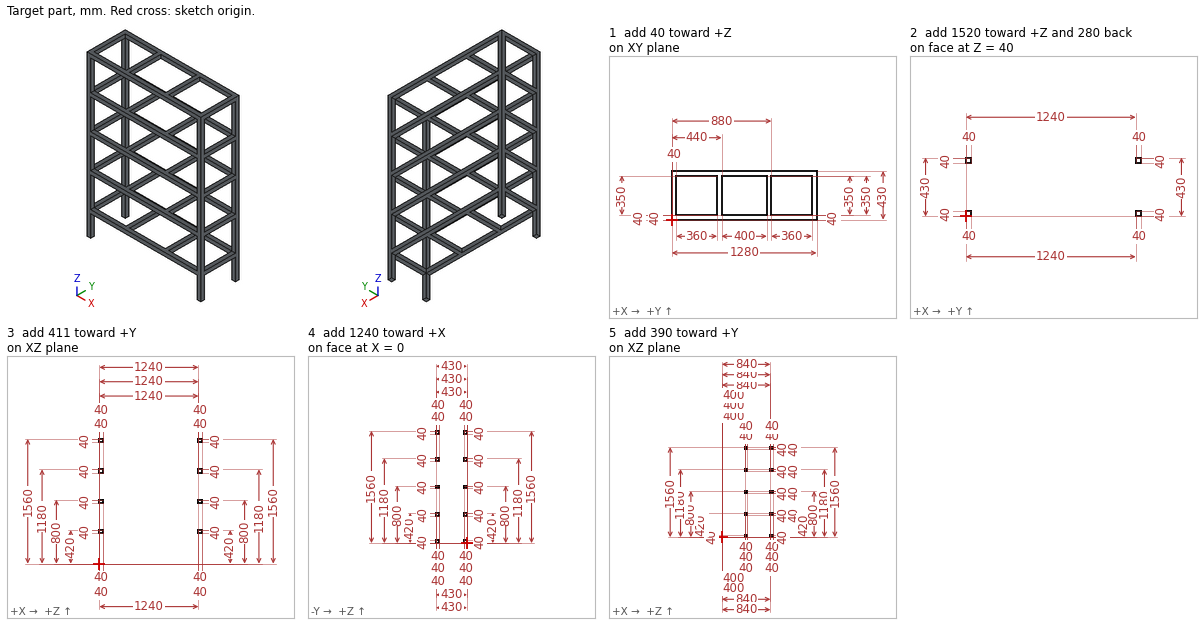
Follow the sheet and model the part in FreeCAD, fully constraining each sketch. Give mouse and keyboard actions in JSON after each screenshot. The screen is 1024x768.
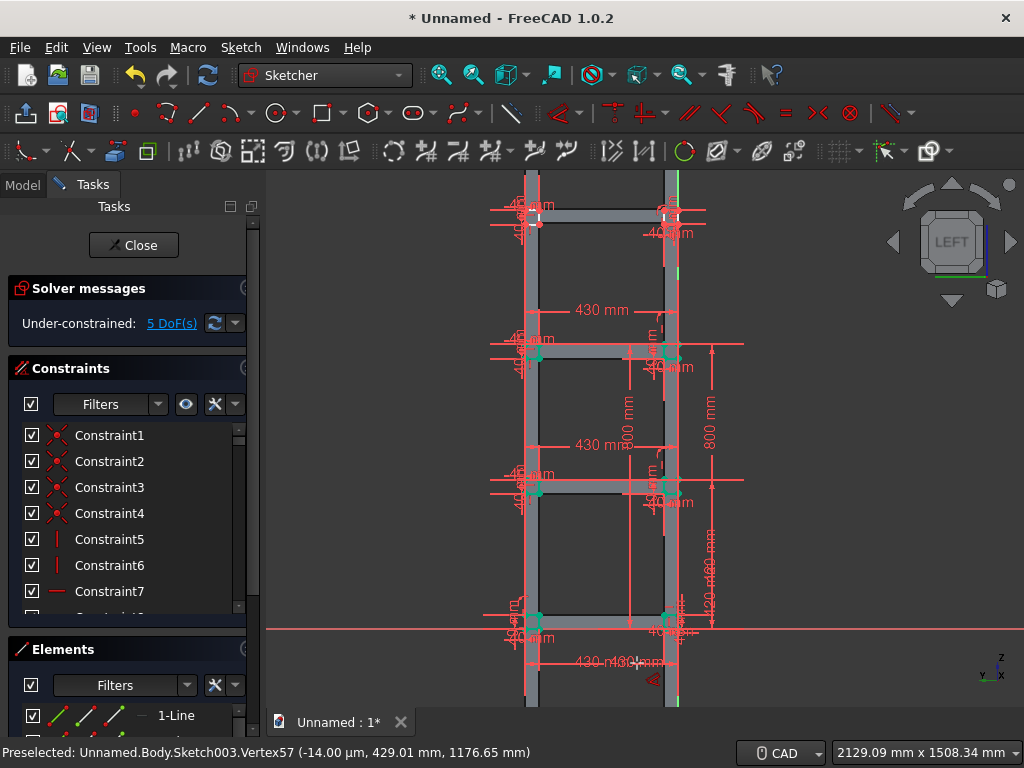
{"action": "scroll", "coordinate": [525, 615], "scroll_direction": "down", "scroll_amount": 2}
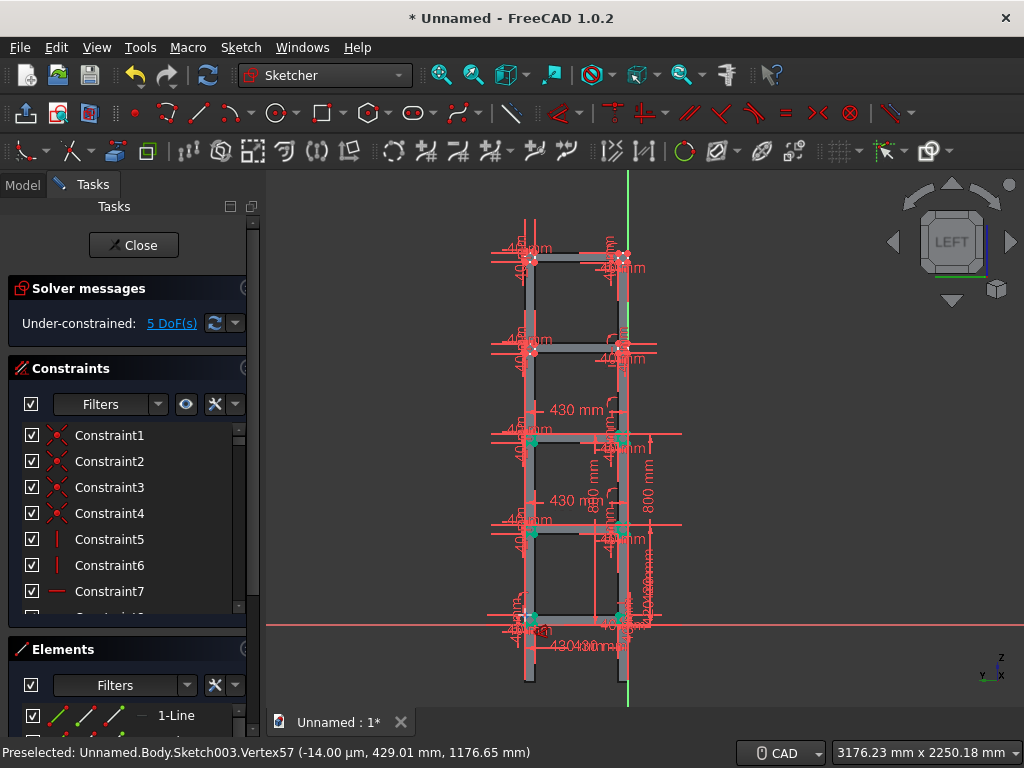
{"action": "scroll", "coordinate": [525, 253], "scroll_direction": "up", "scroll_amount": 2}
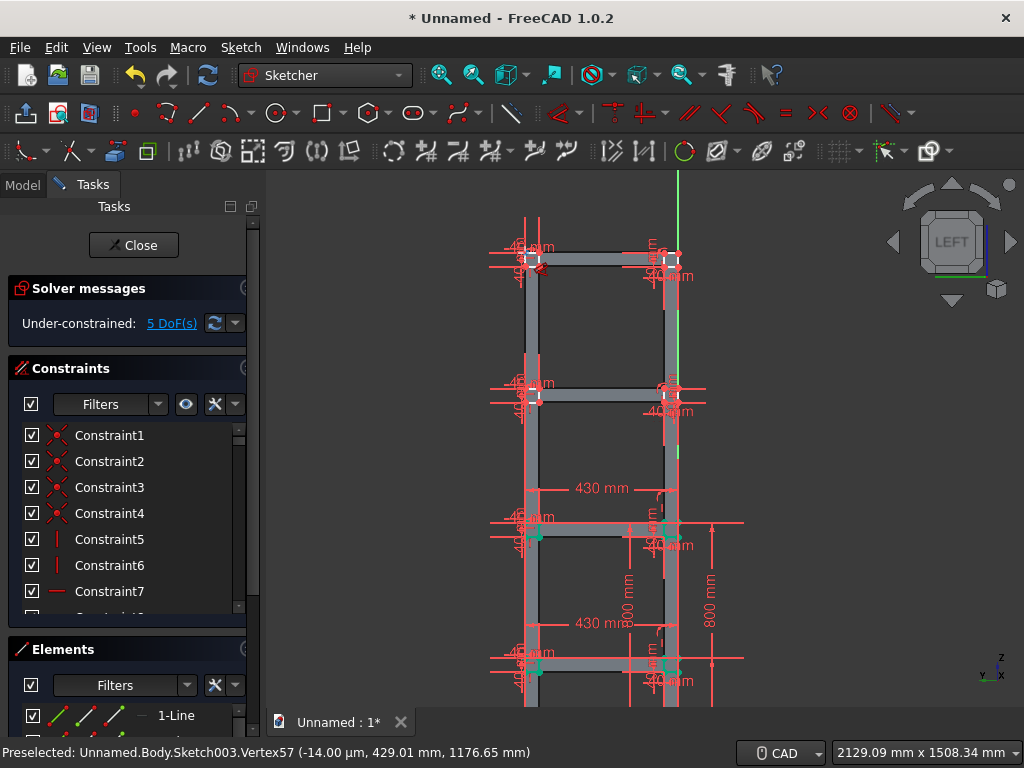
{"action": "left_click", "coordinate": [525, 253]}
{"action": "left_click", "coordinate": [602, 219]}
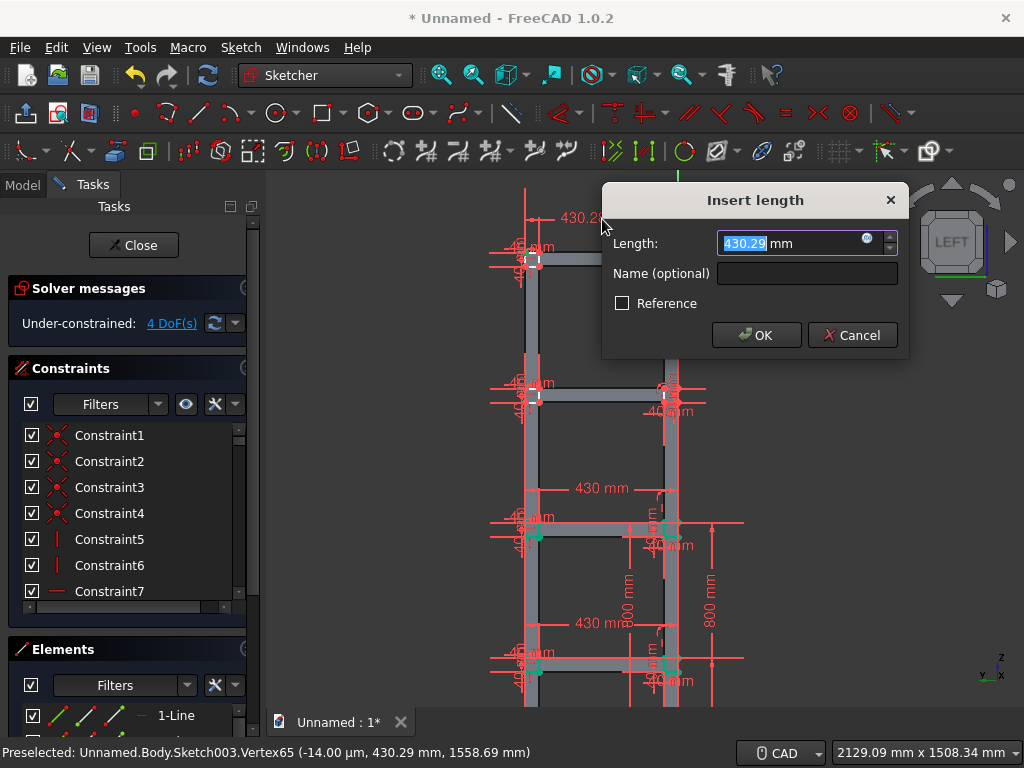
{"action": "type", "text": "430"}
{"action": "key", "text": "Return"}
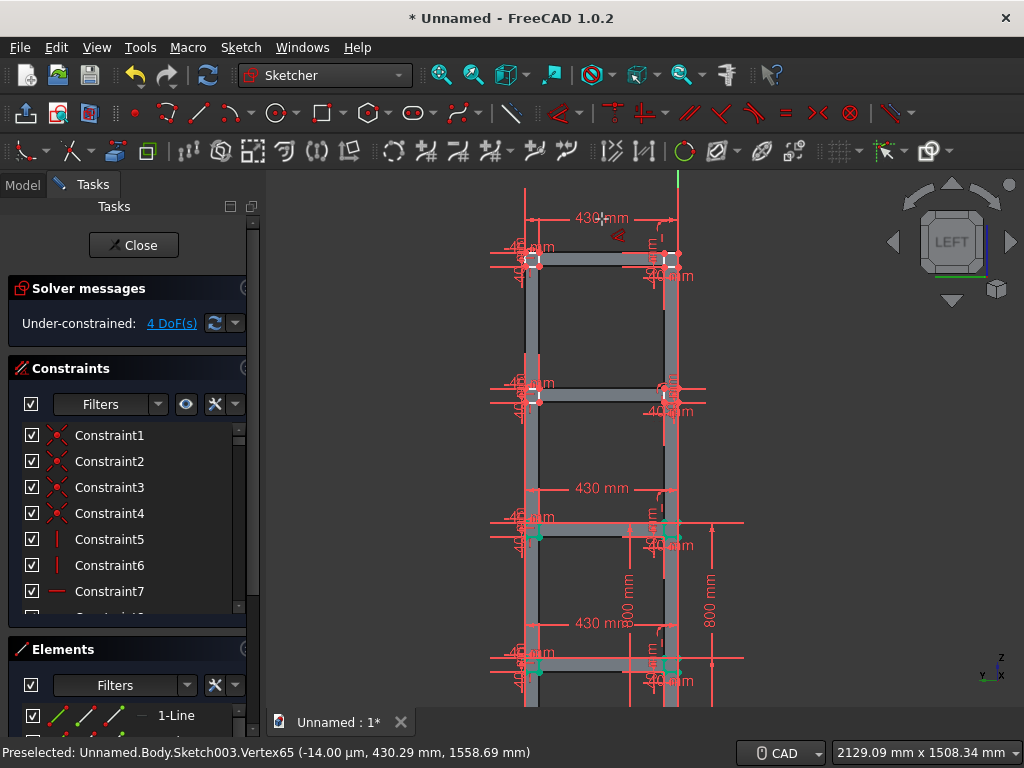
{"action": "left_click", "coordinate": [664, 389]}
{"action": "left_click", "coordinate": [712, 467]}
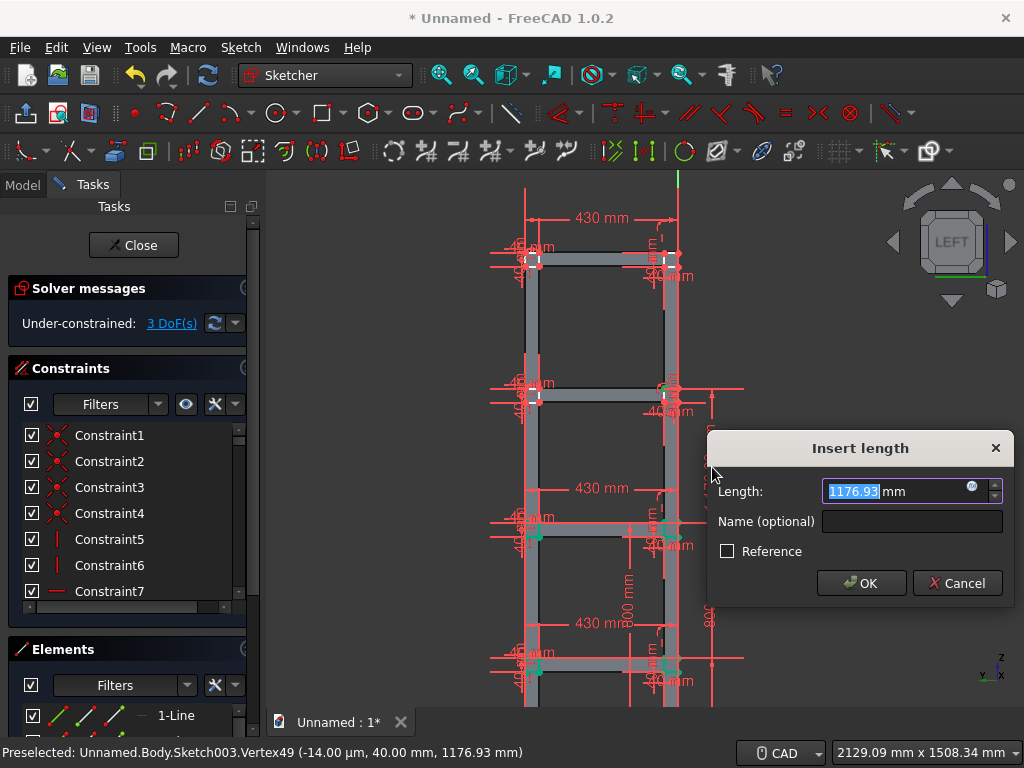
{"action": "type", "text": "1180"}
{"action": "key", "text": "Return"}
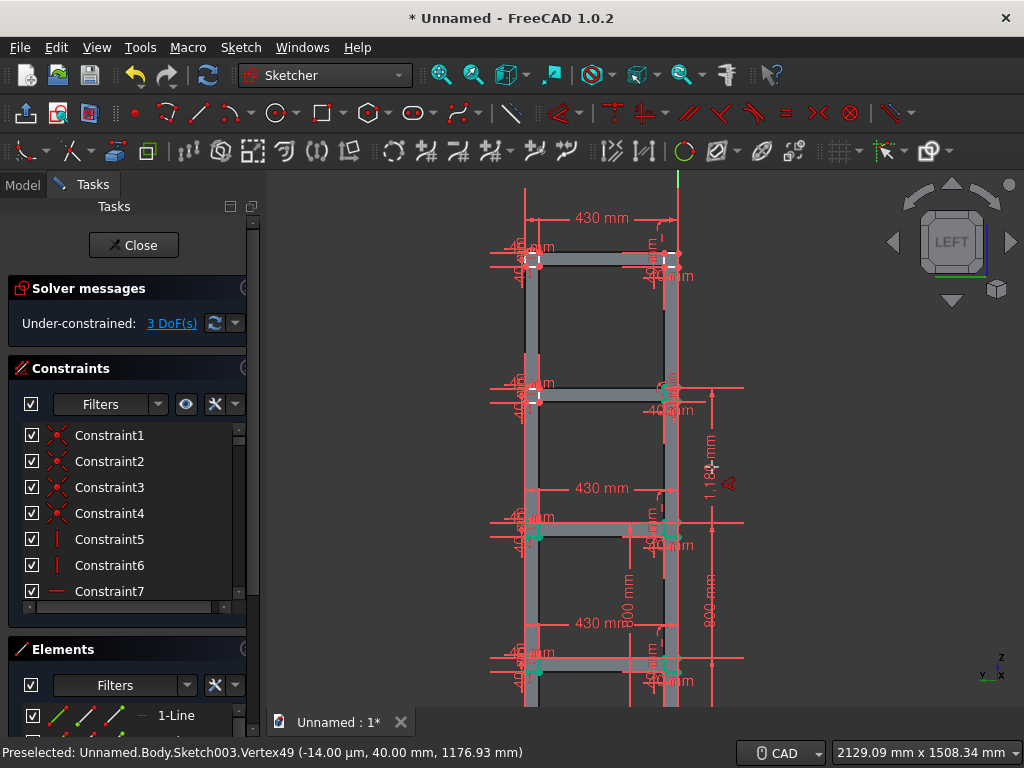
{"action": "left_click", "coordinate": [525, 389]}
{"action": "left_click", "coordinate": [712, 635]}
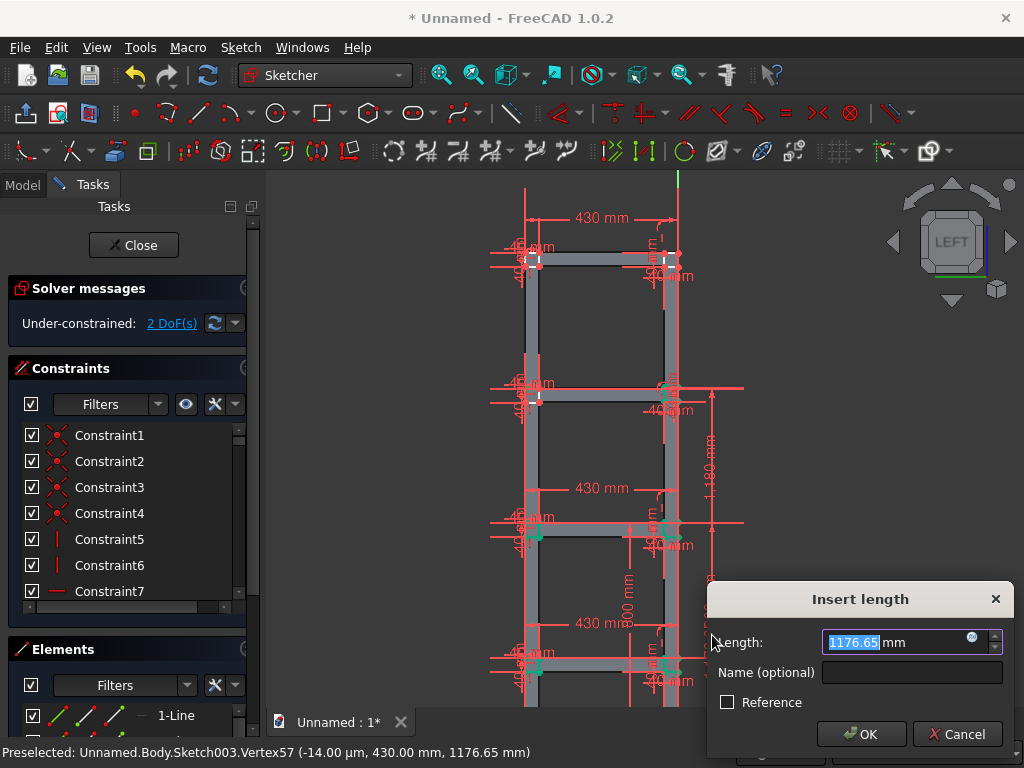
{"action": "type", "text": "1180"}
{"action": "key", "text": "Return"}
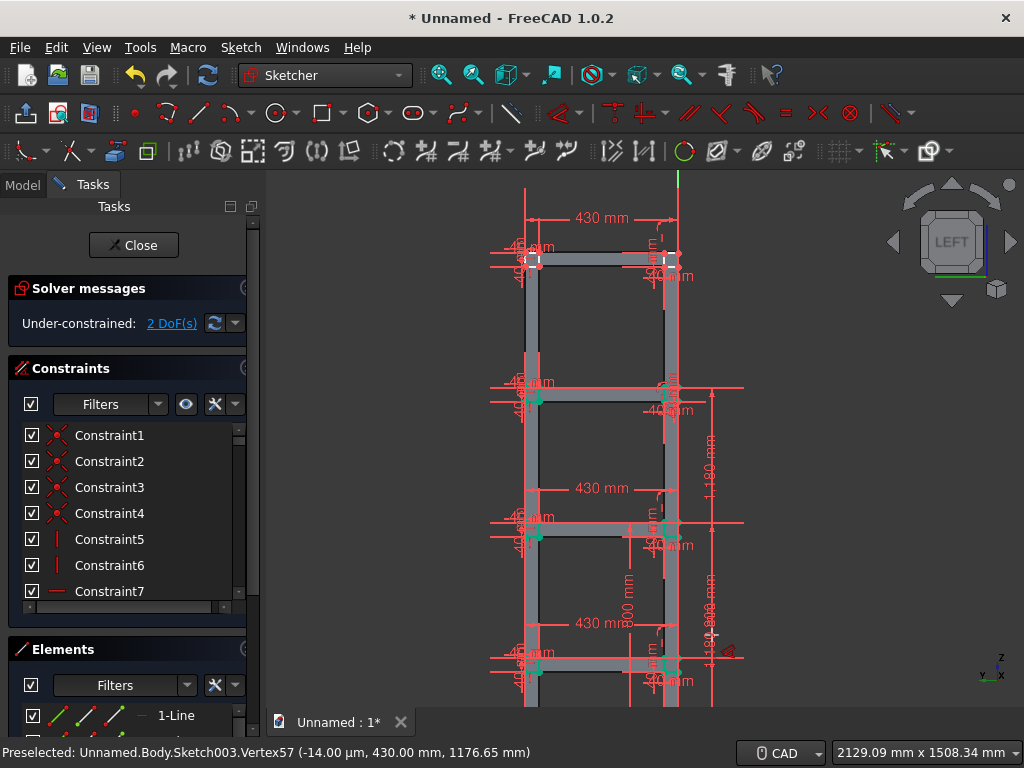
{"action": "left_click", "coordinate": [525, 253]}
{"action": "left_click", "coordinate": [712, 368]}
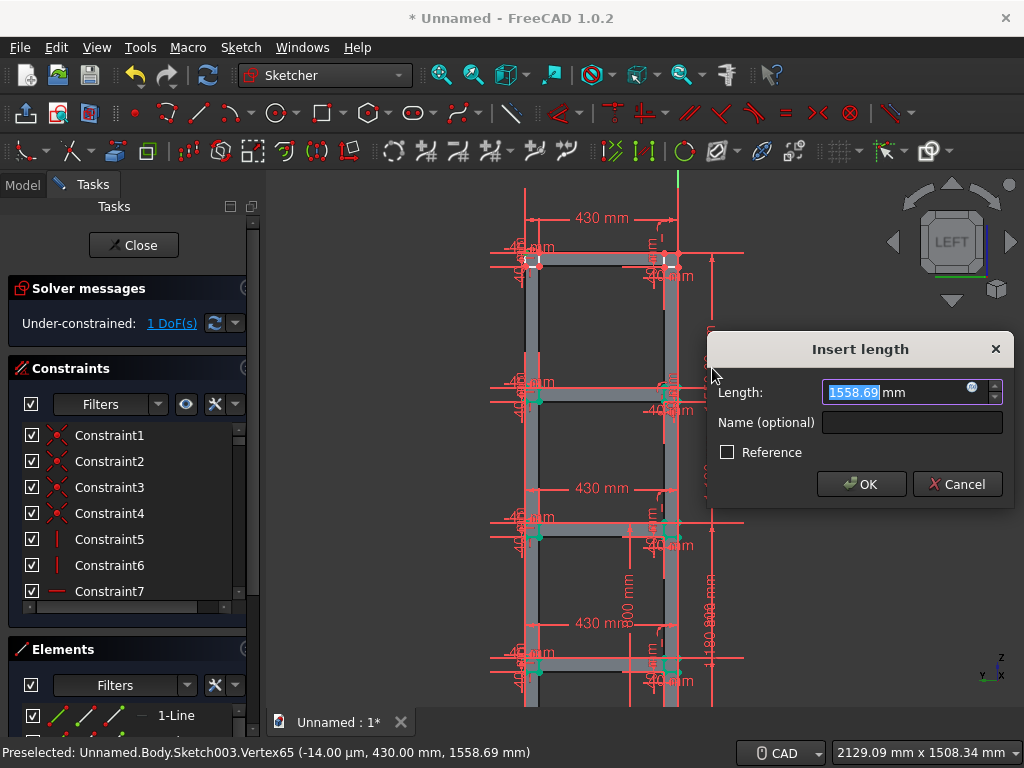
{"action": "type", "text": "1560"}
{"action": "key", "text": "Return"}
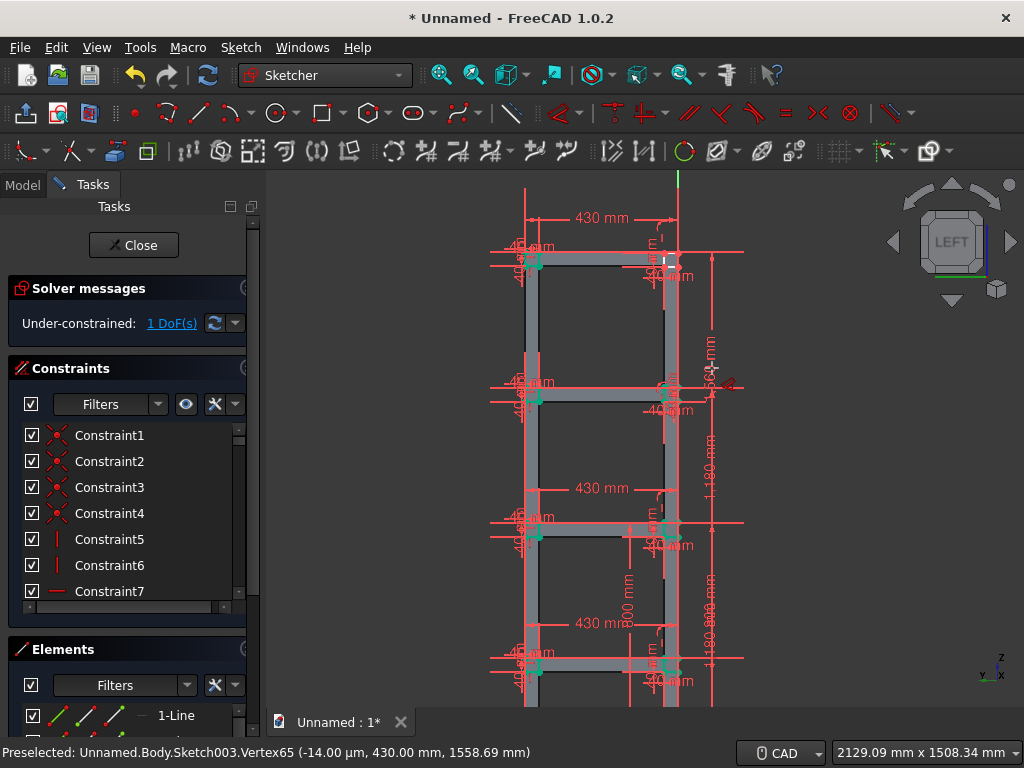
{"action": "left_click", "coordinate": [664, 253]}
{"action": "left_click", "coordinate": [712, 317]}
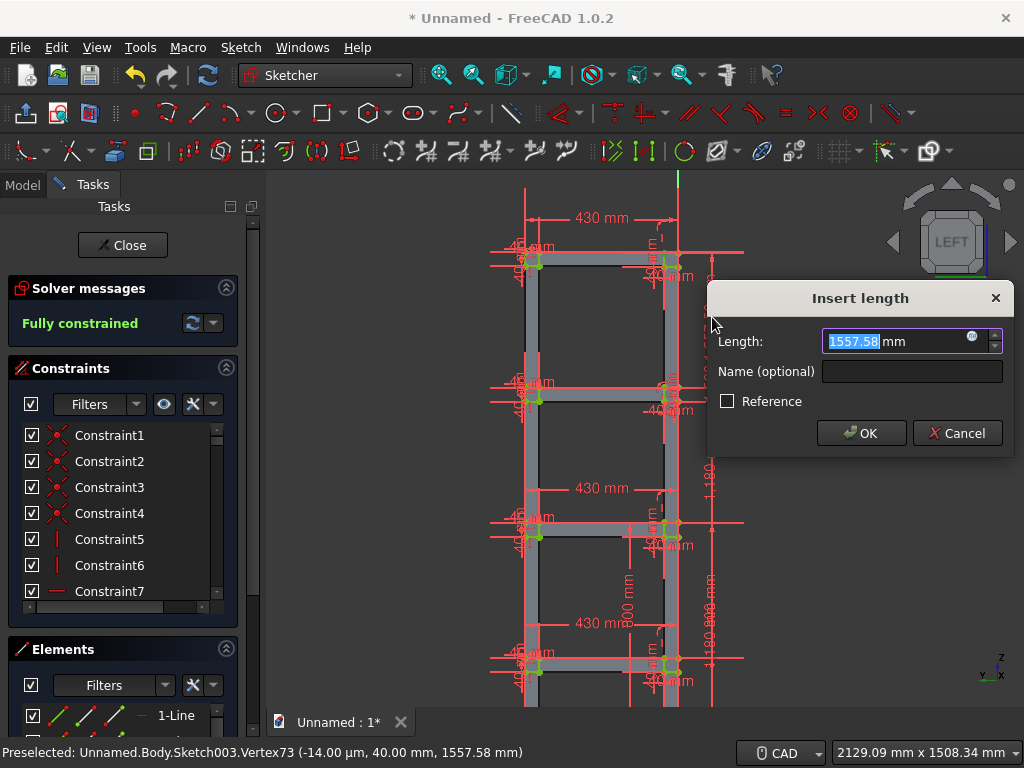
{"action": "type", "text": "1560"}
{"action": "key", "text": "Return"}
{"action": "key", "text": "Escape"}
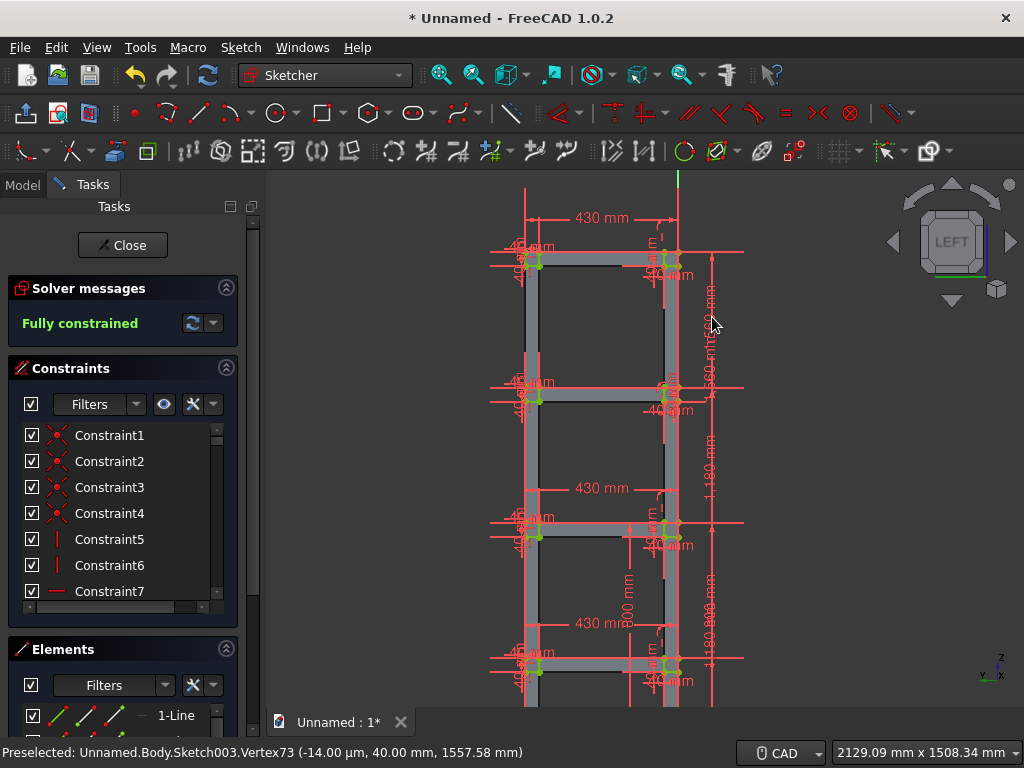
{"action": "left_click", "coordinate": [123, 245]}